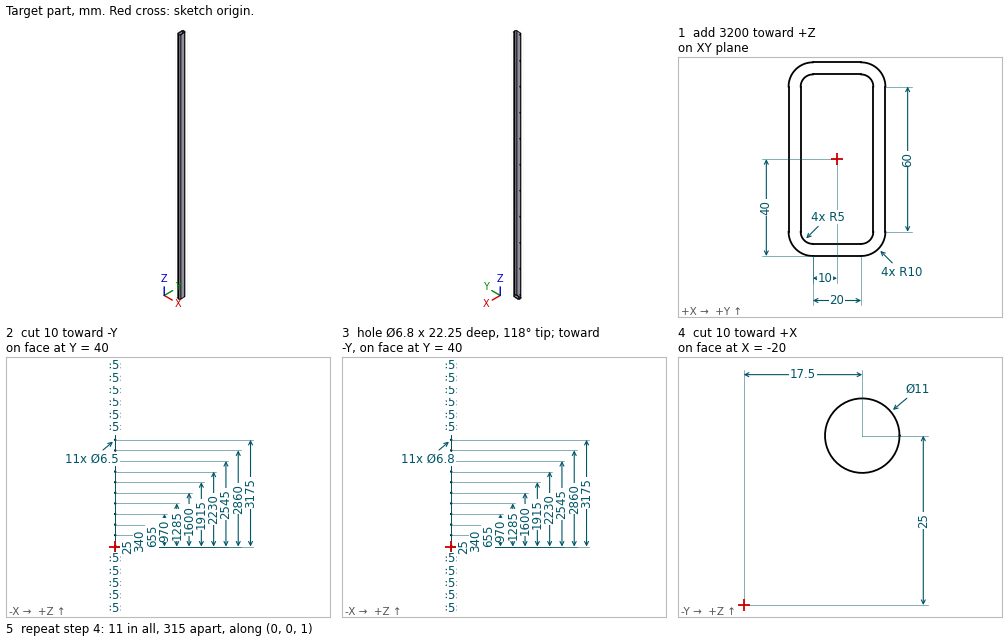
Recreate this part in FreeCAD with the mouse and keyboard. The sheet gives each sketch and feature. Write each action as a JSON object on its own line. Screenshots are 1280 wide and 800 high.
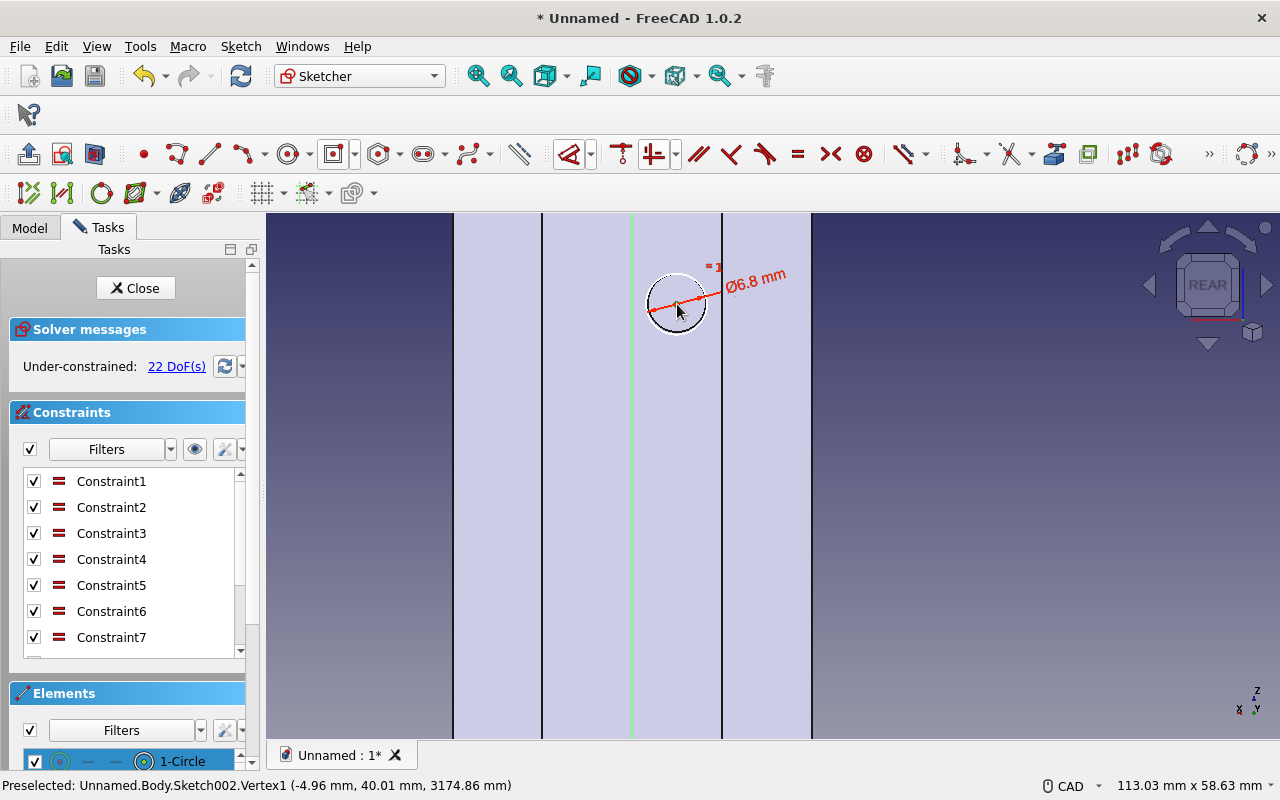
{"action": "key", "text": "l"}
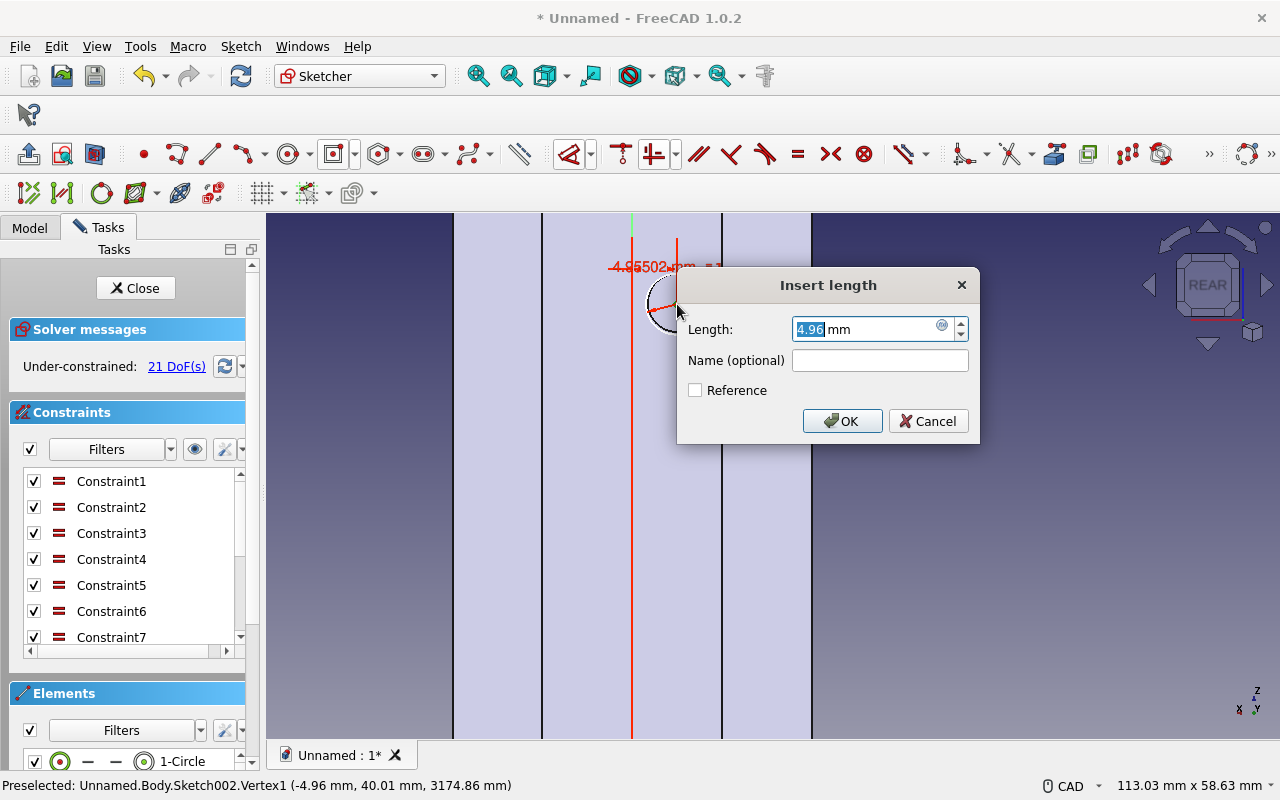
{"action": "type", "text": "5"}
{"action": "key", "text": "Return"}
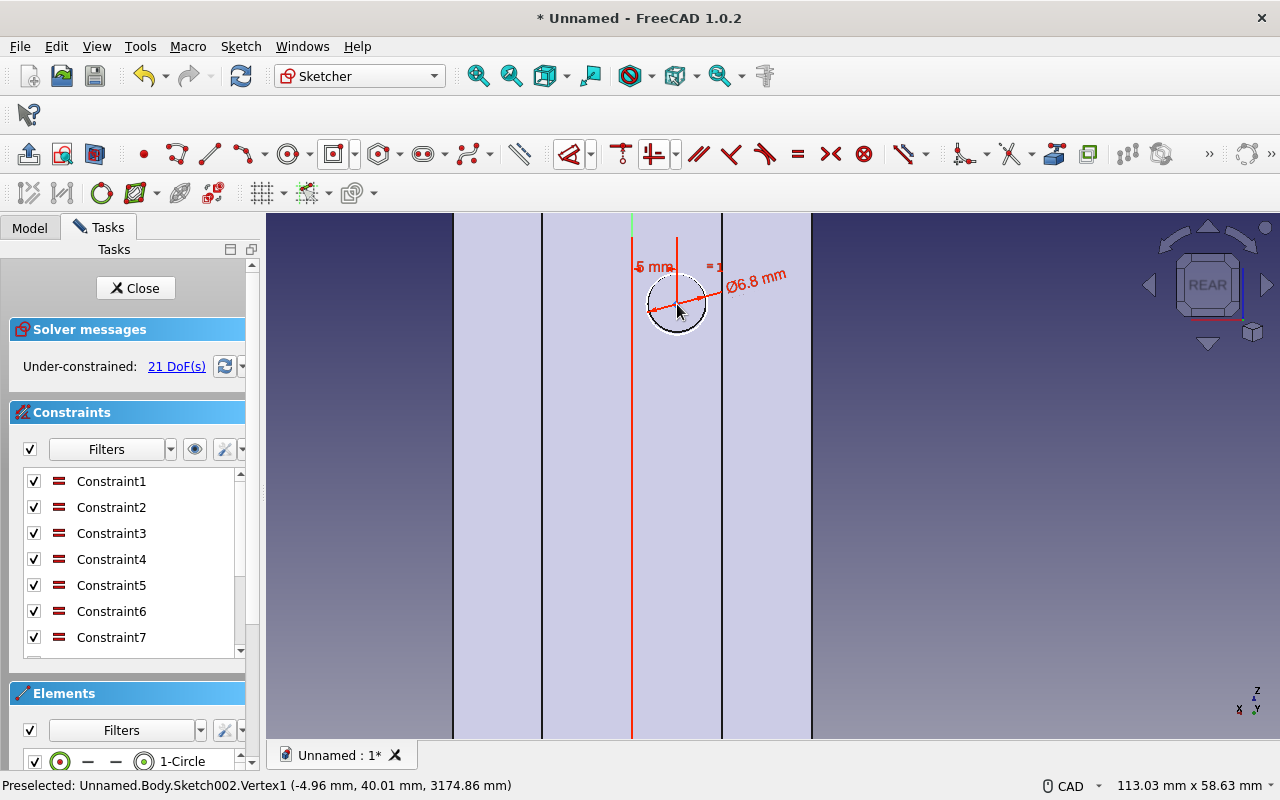
{"action": "scroll", "coordinate": [704, 476], "scroll_direction": "down", "scroll_amount": 15}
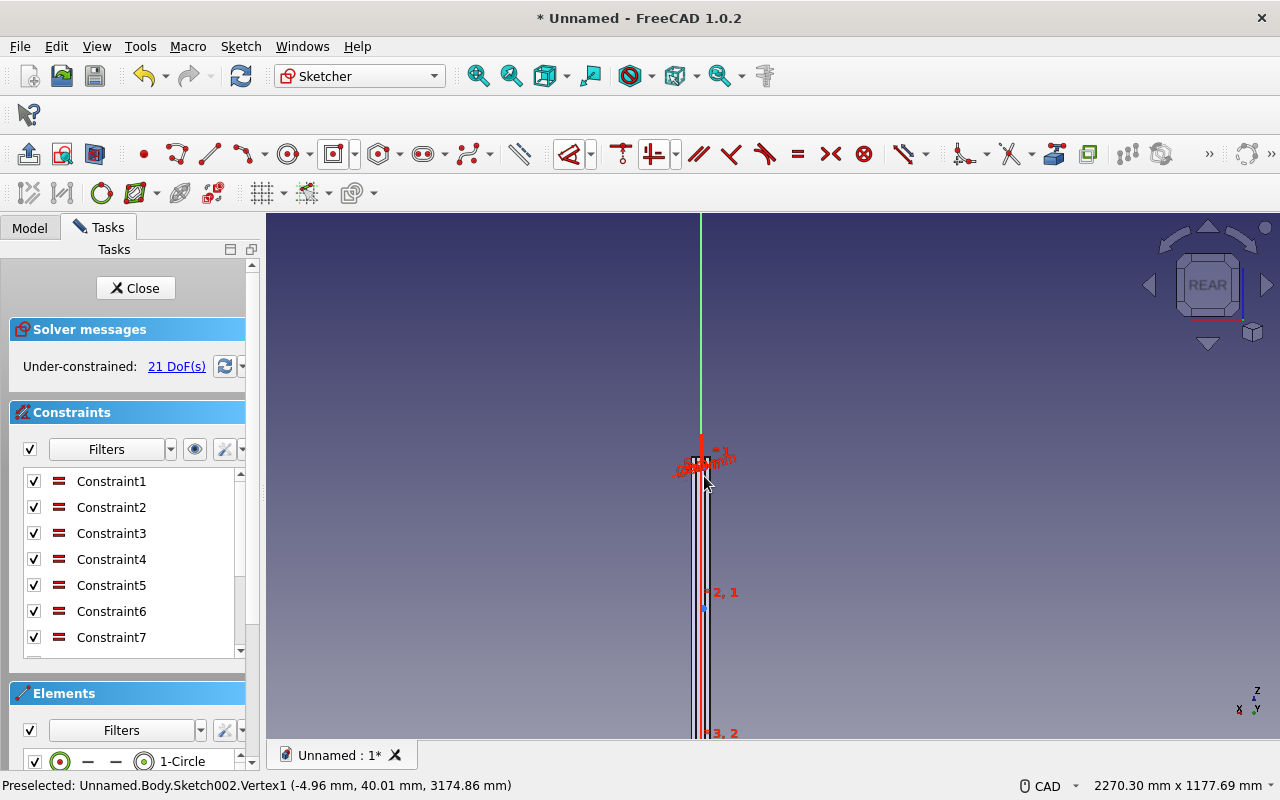
{"action": "scroll", "coordinate": [705, 247], "scroll_direction": "down", "scroll_amount": 7}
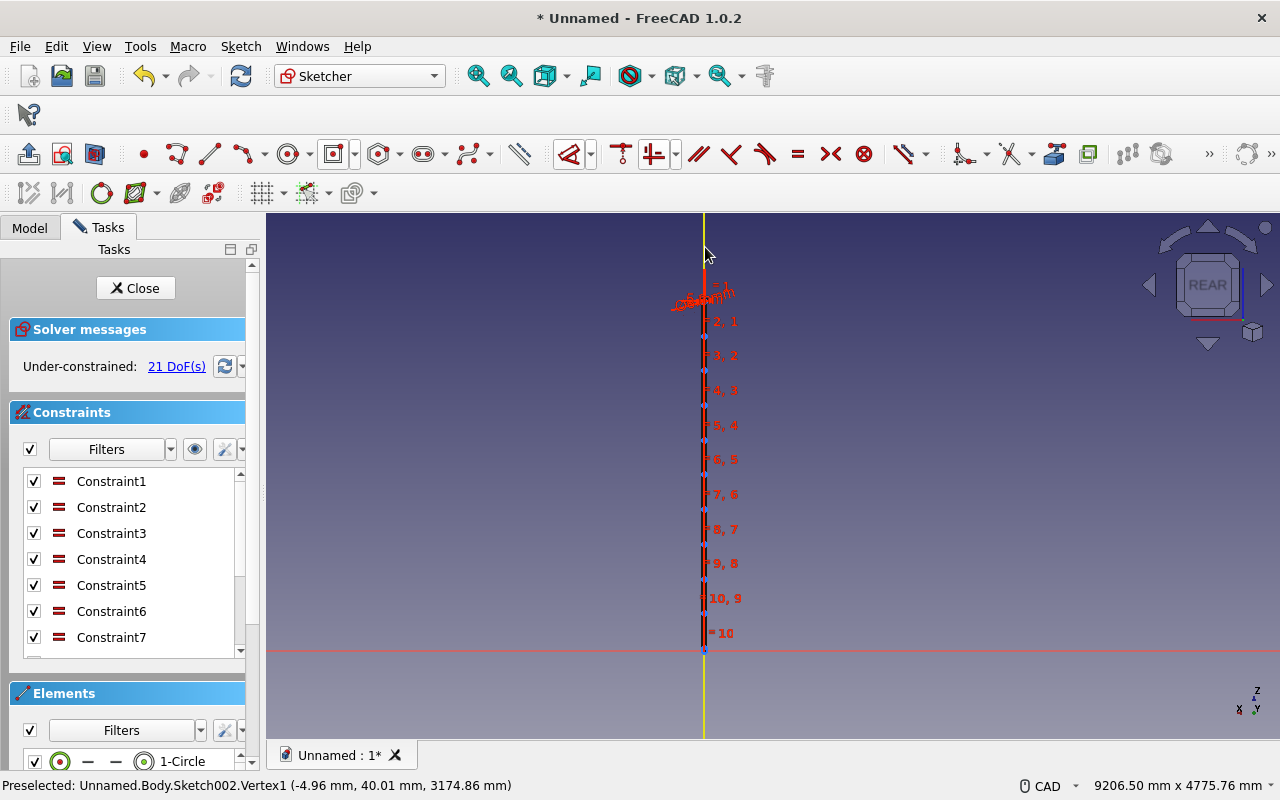
{"action": "scroll", "coordinate": [705, 336], "scroll_direction": "up", "scroll_amount": 22}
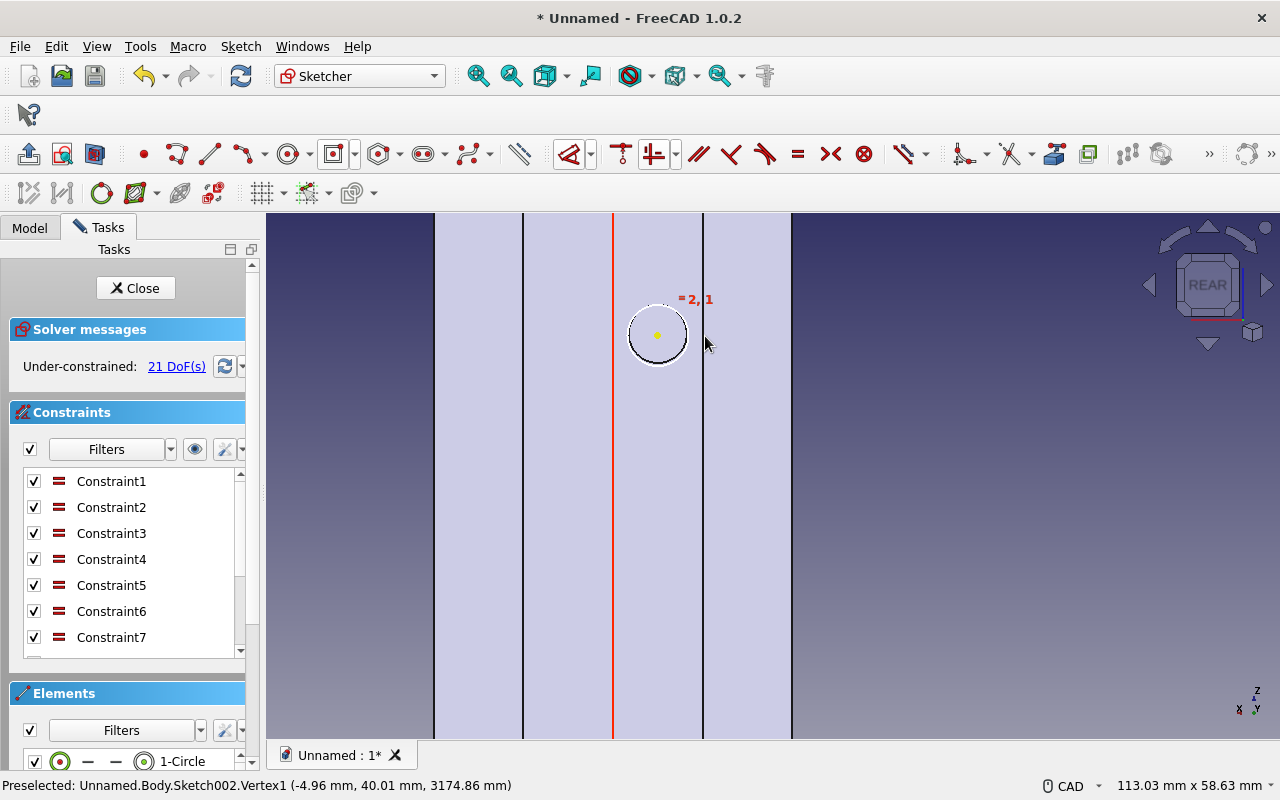
{"action": "left_click", "coordinate": [658, 336]}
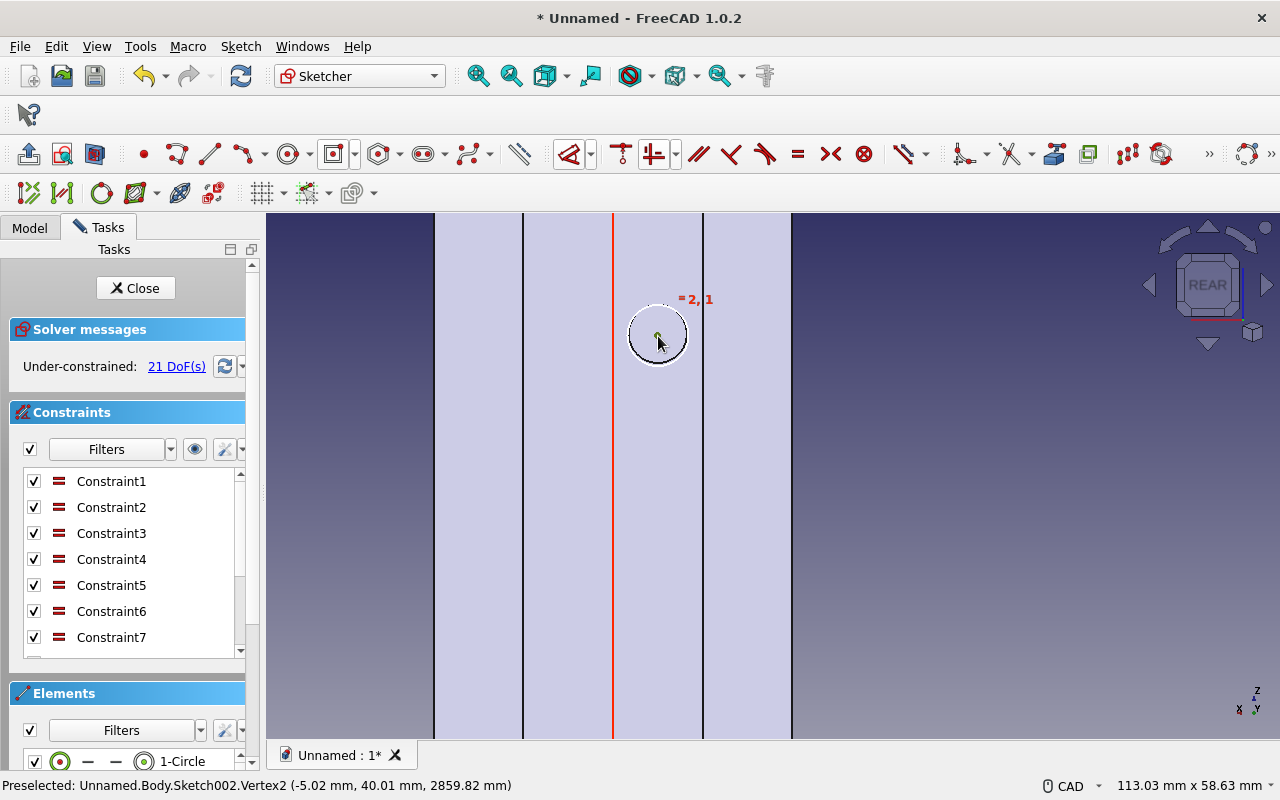
{"action": "left_click", "coordinate": [590, 154]}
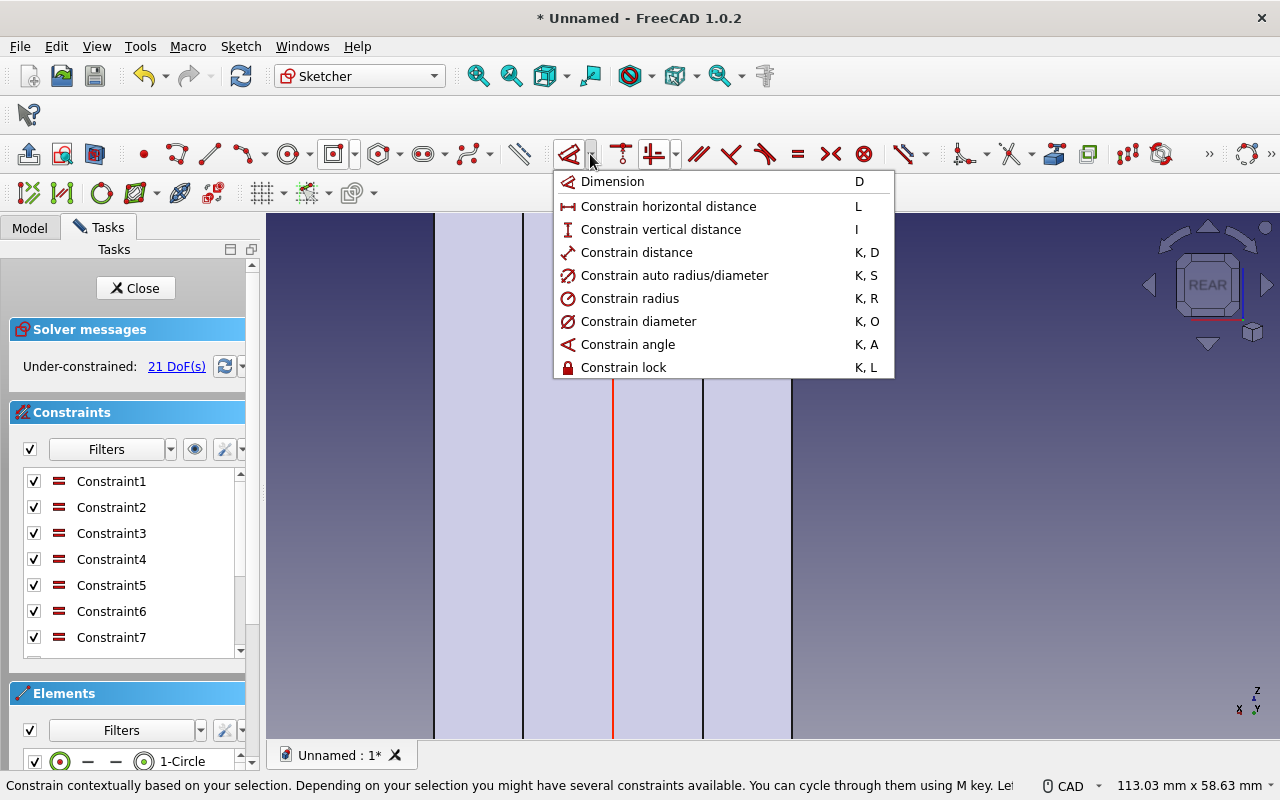
{"action": "left_click", "coordinate": [724, 206]}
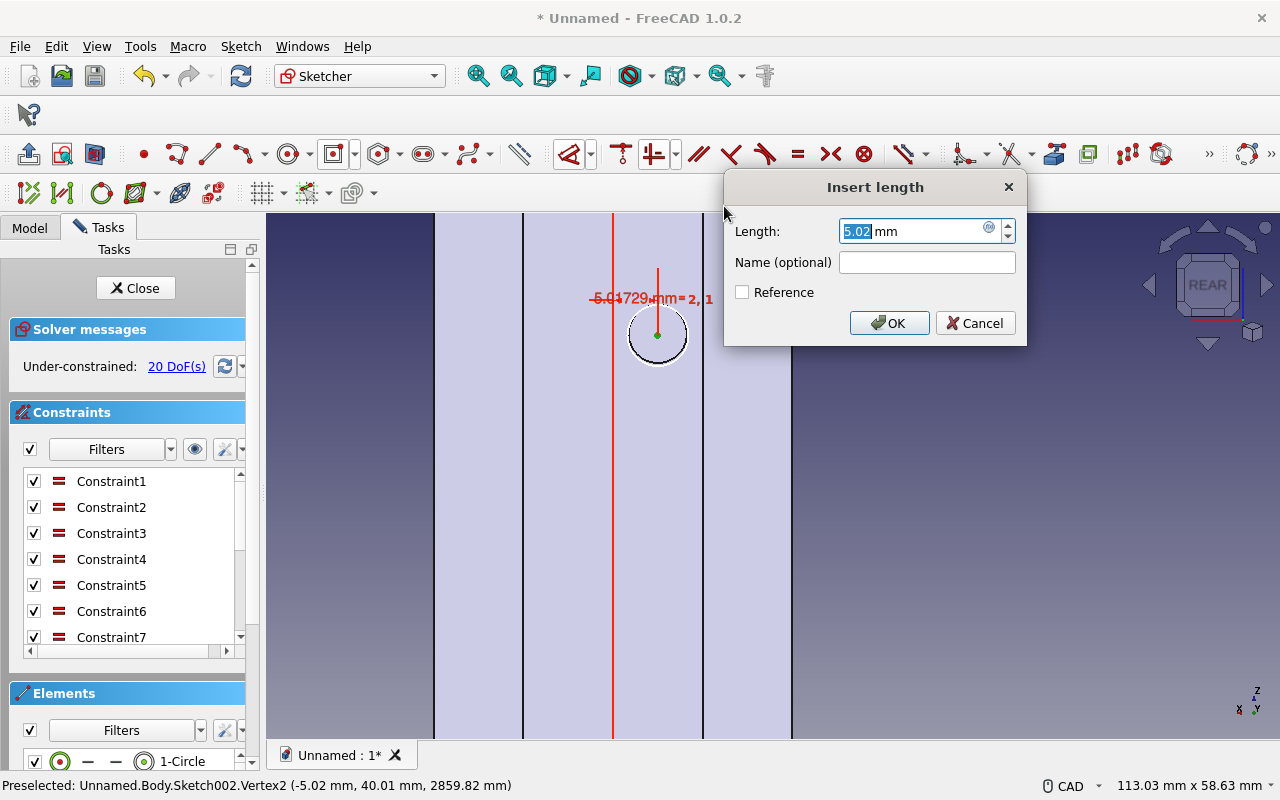
{"action": "type", "text": "5"}
{"action": "key", "text": "Return"}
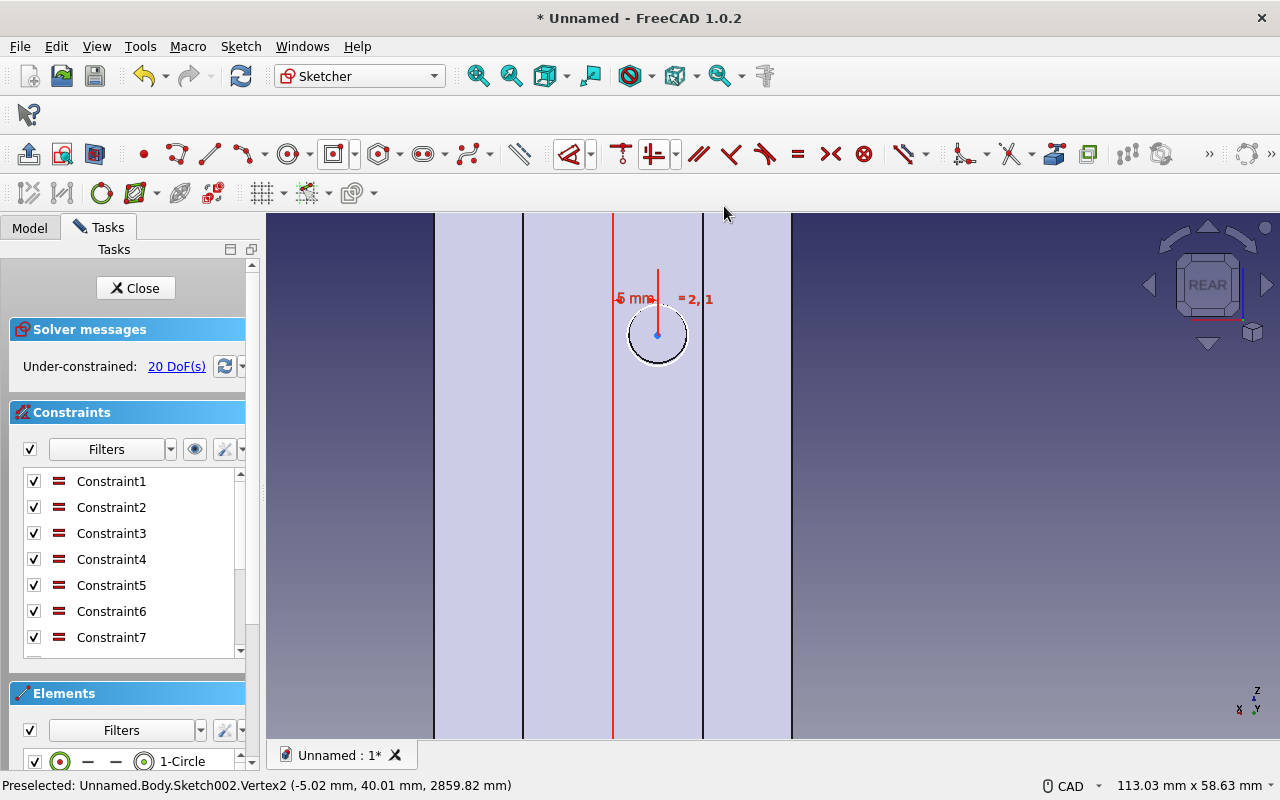
{"action": "scroll", "coordinate": [704, 476], "scroll_direction": "down", "scroll_amount": 15}